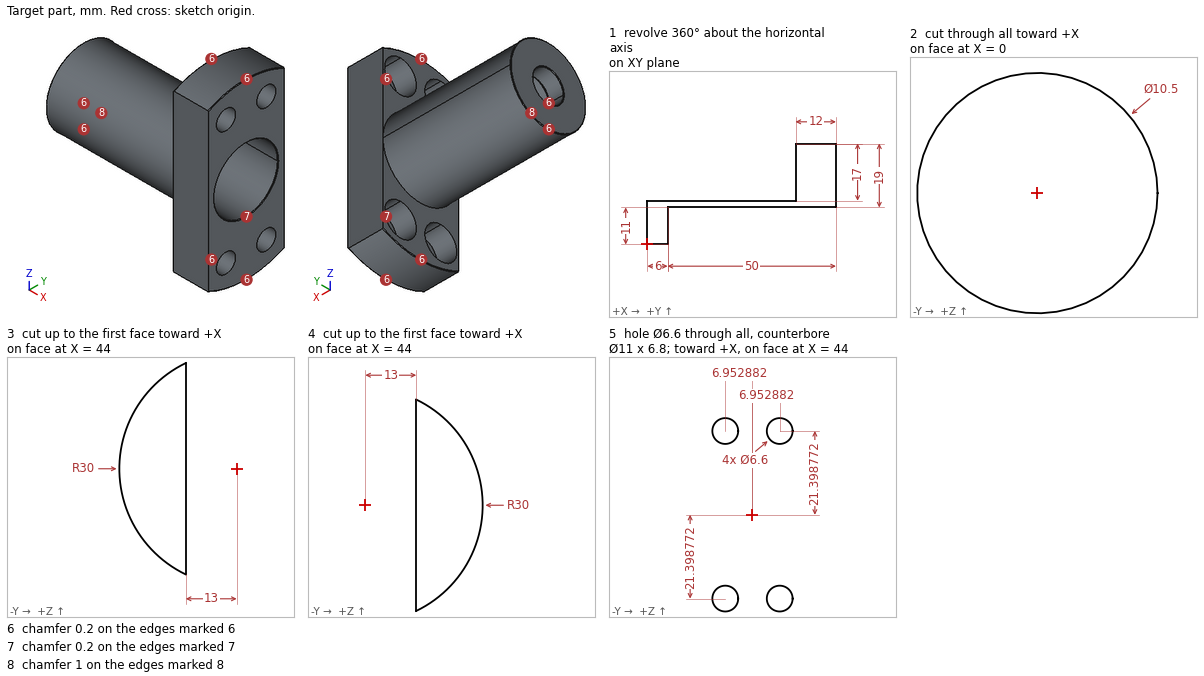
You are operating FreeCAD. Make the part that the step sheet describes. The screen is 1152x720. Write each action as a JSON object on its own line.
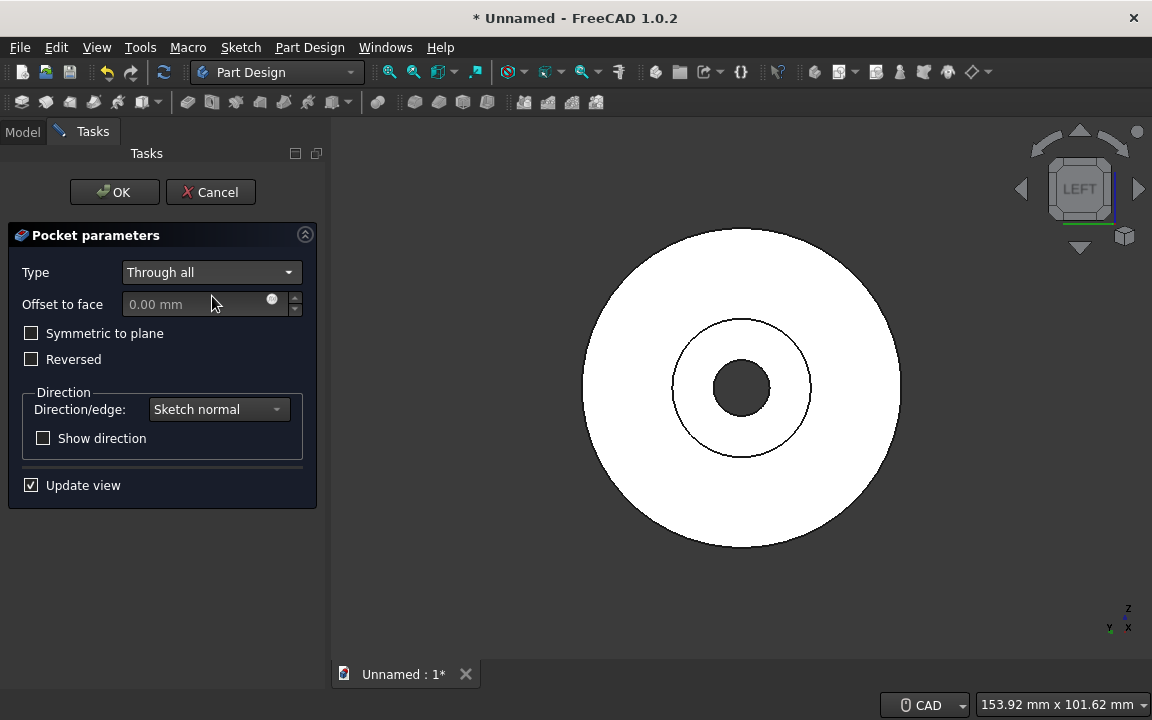
{"action": "left_click", "coordinate": [115, 192]}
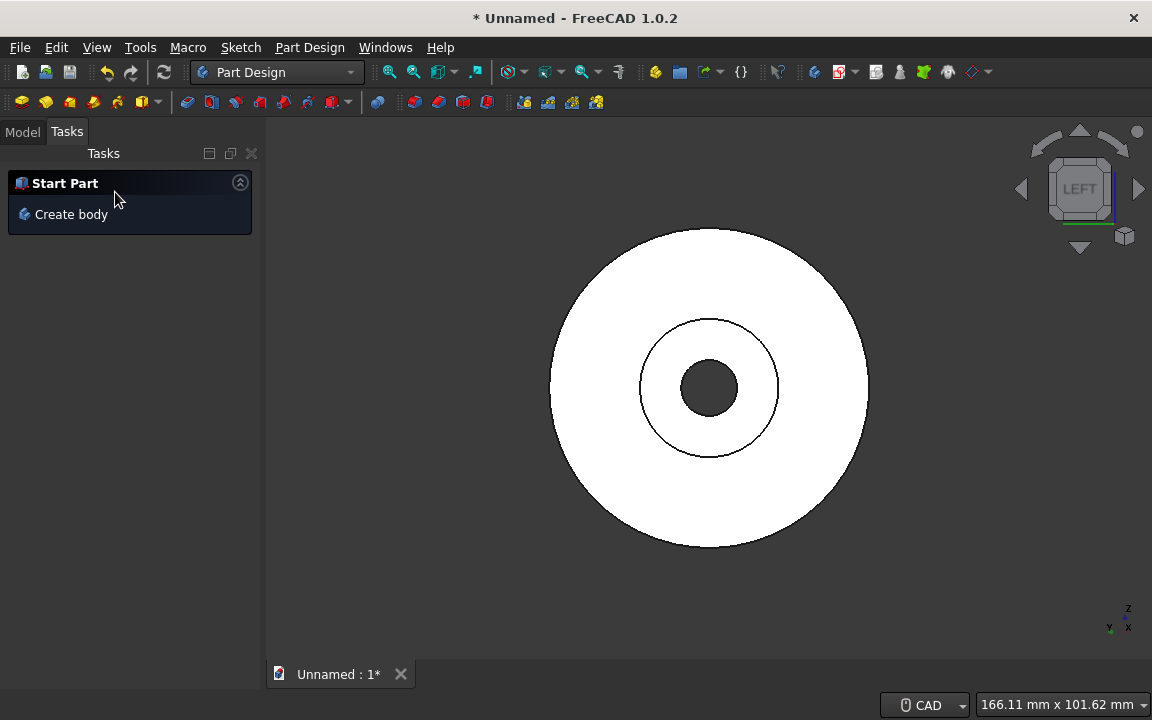
{"action": "left_click", "coordinate": [755, 296]}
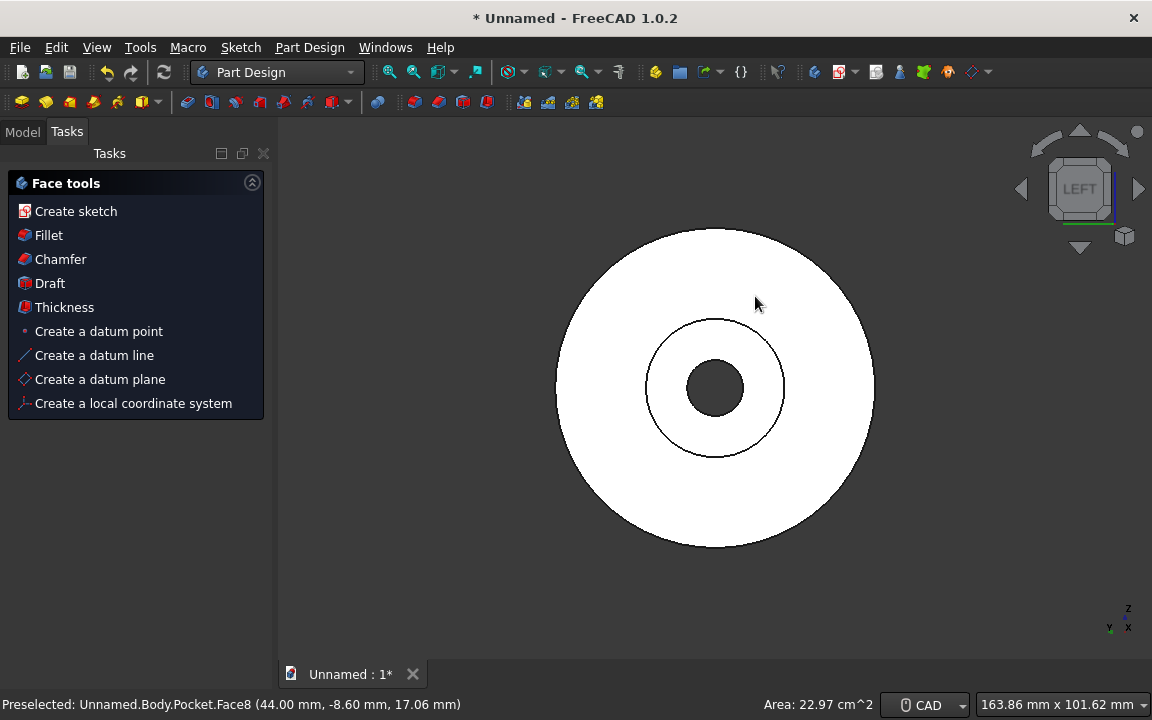
{"action": "left_click", "coordinate": [840, 72]}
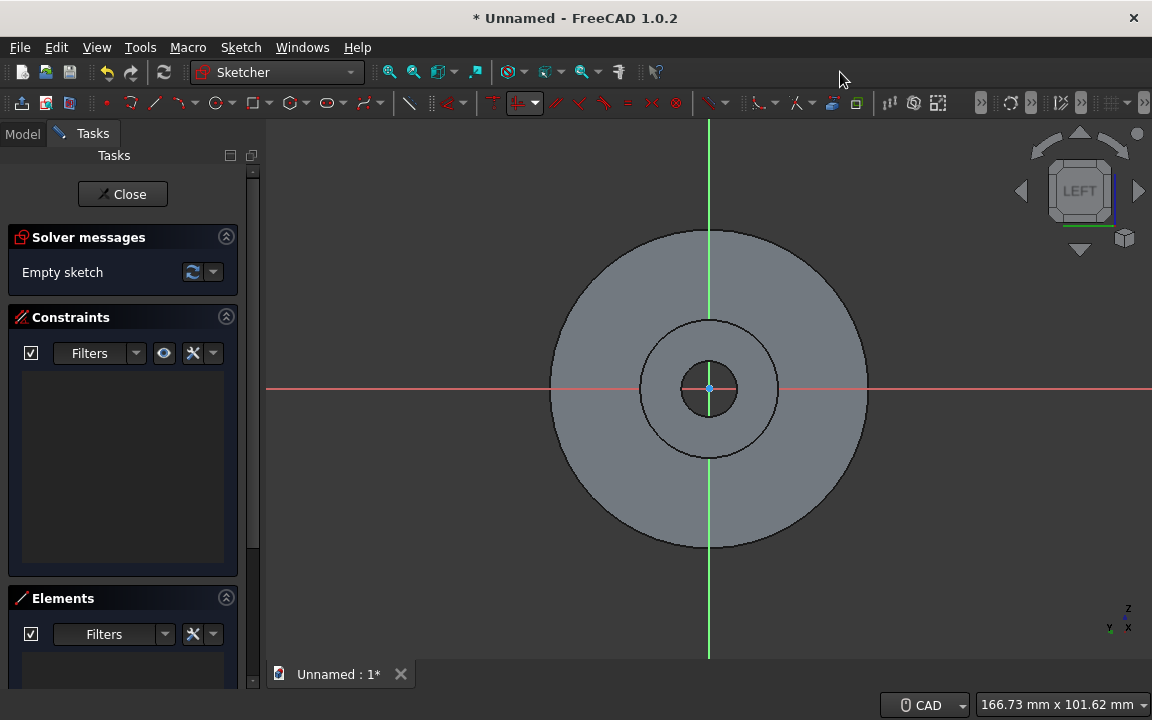
{"action": "left_click", "coordinate": [156, 104]}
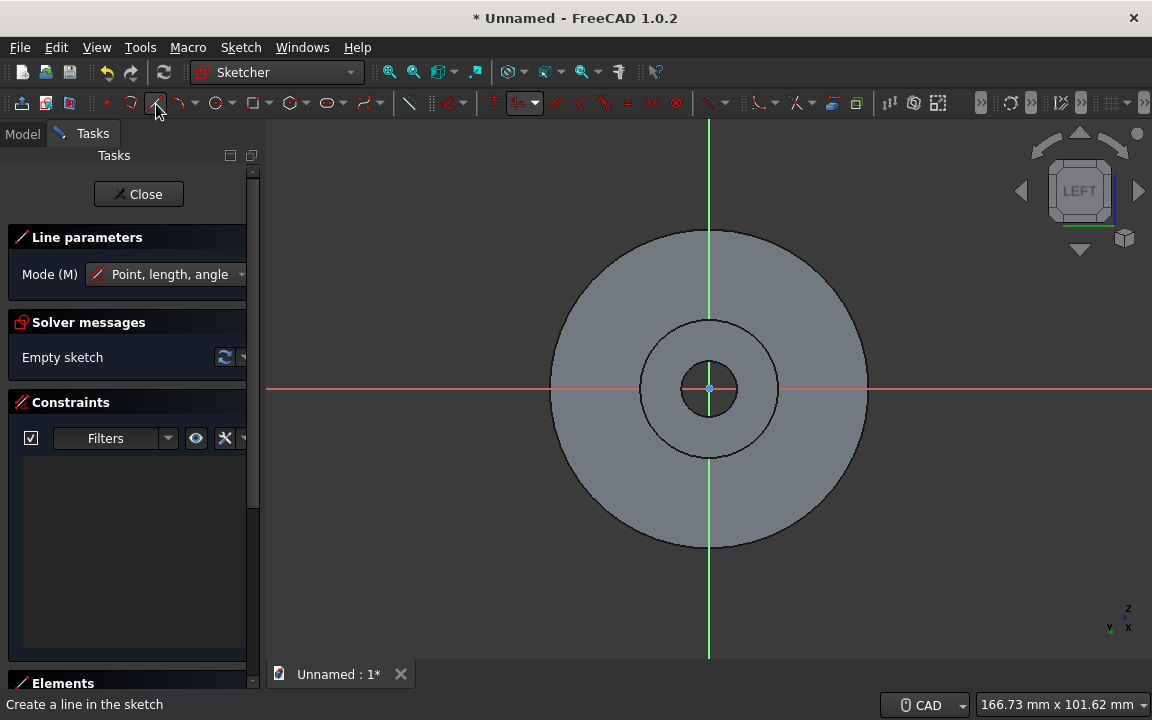
{"action": "left_click", "coordinate": [640, 533]}
{"action": "left_click", "coordinate": [640, 245]}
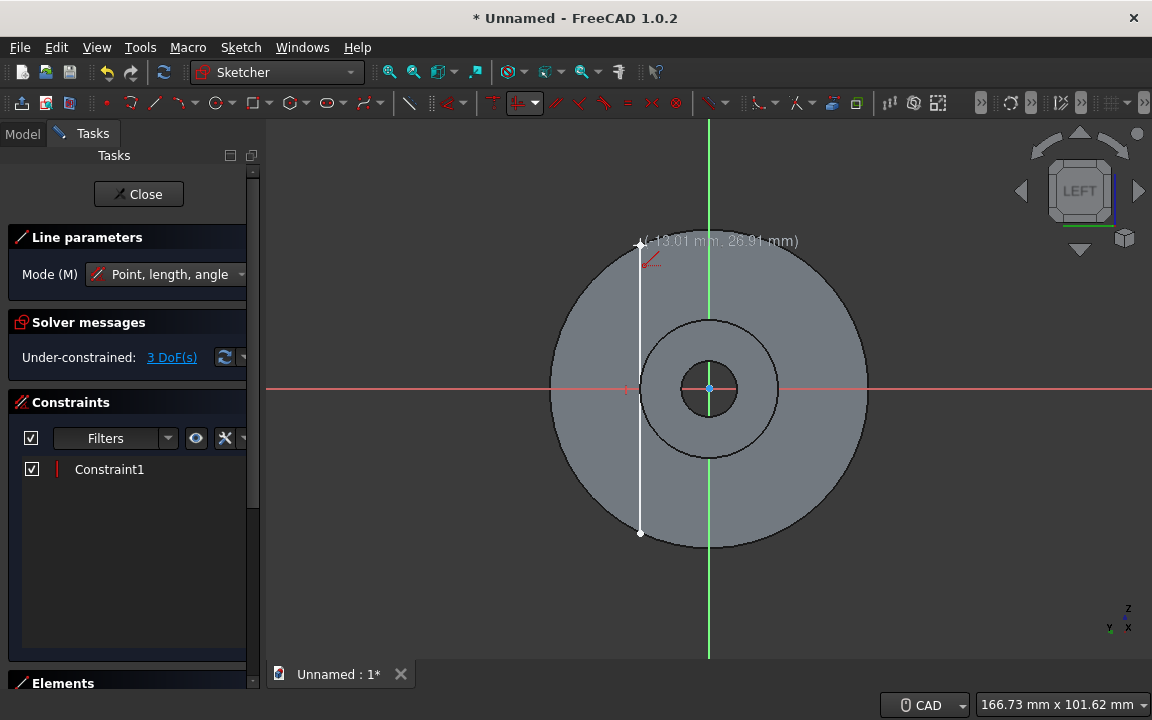
{"action": "left_click", "coordinate": [180, 104]}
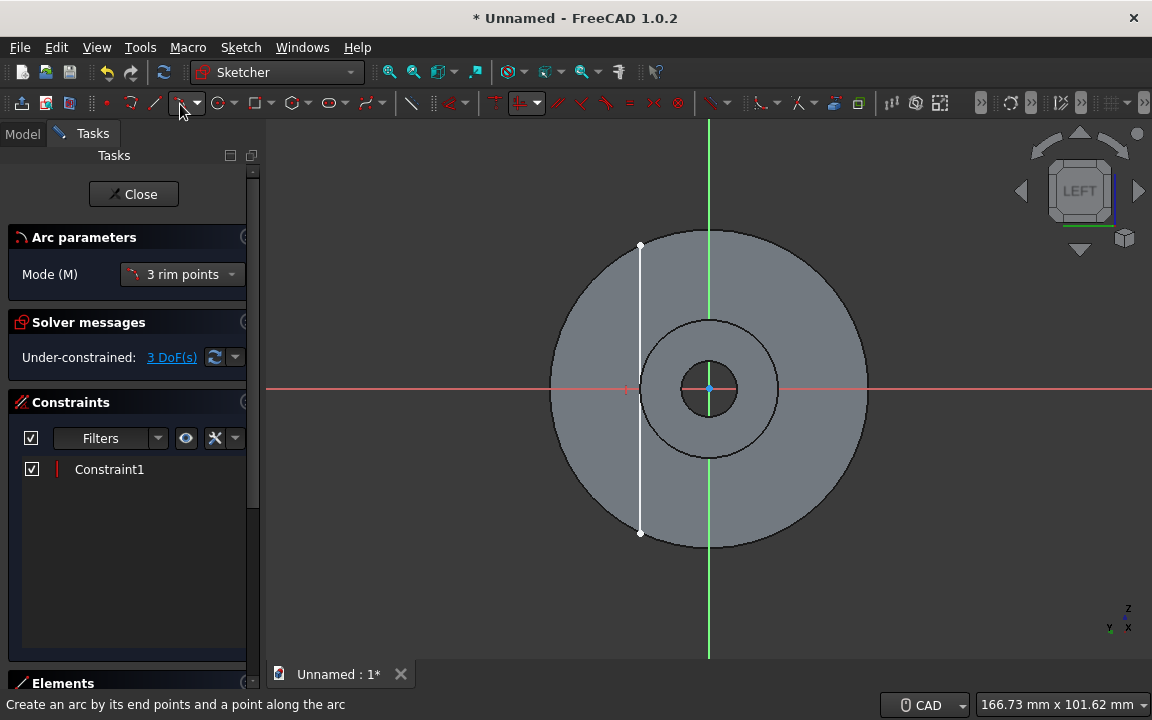
{"action": "left_click", "coordinate": [640, 246]}
{"action": "left_click", "coordinate": [640, 534]}
{"action": "left_click", "coordinate": [554, 354]}
{"action": "key", "text": "Escape"}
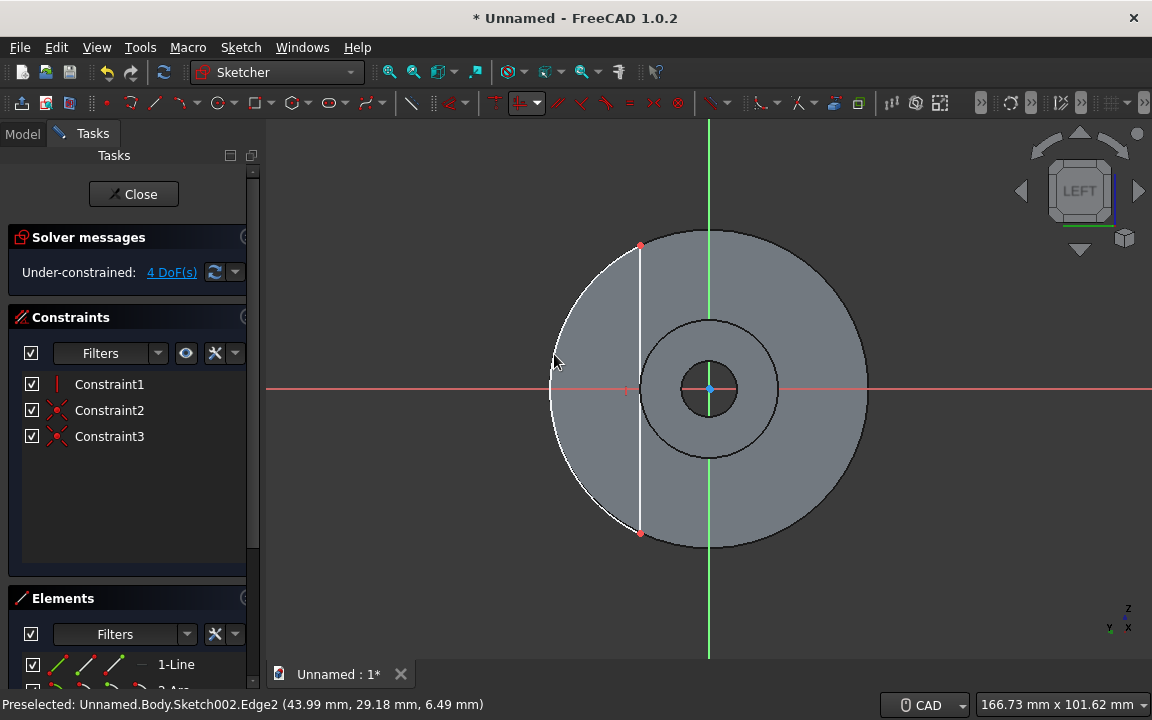
{"action": "left_click_drag", "start_coordinate": [699, 379], "coordinate": [720, 400]}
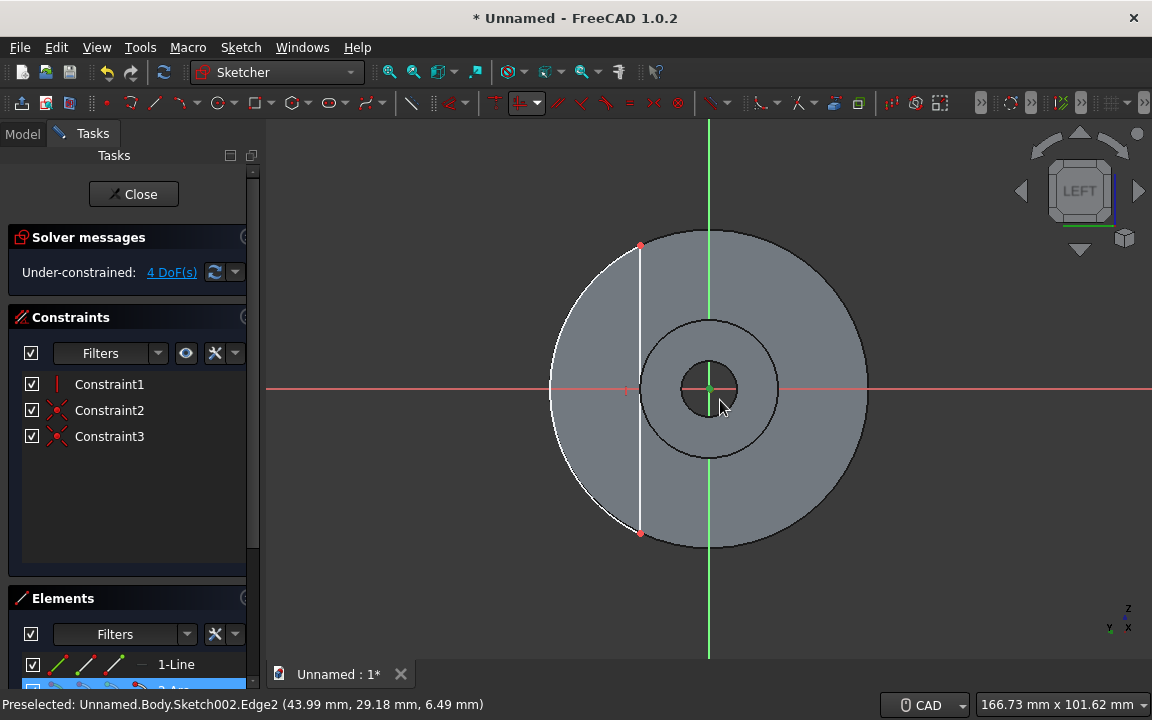
{"action": "left_click", "coordinate": [496, 104]}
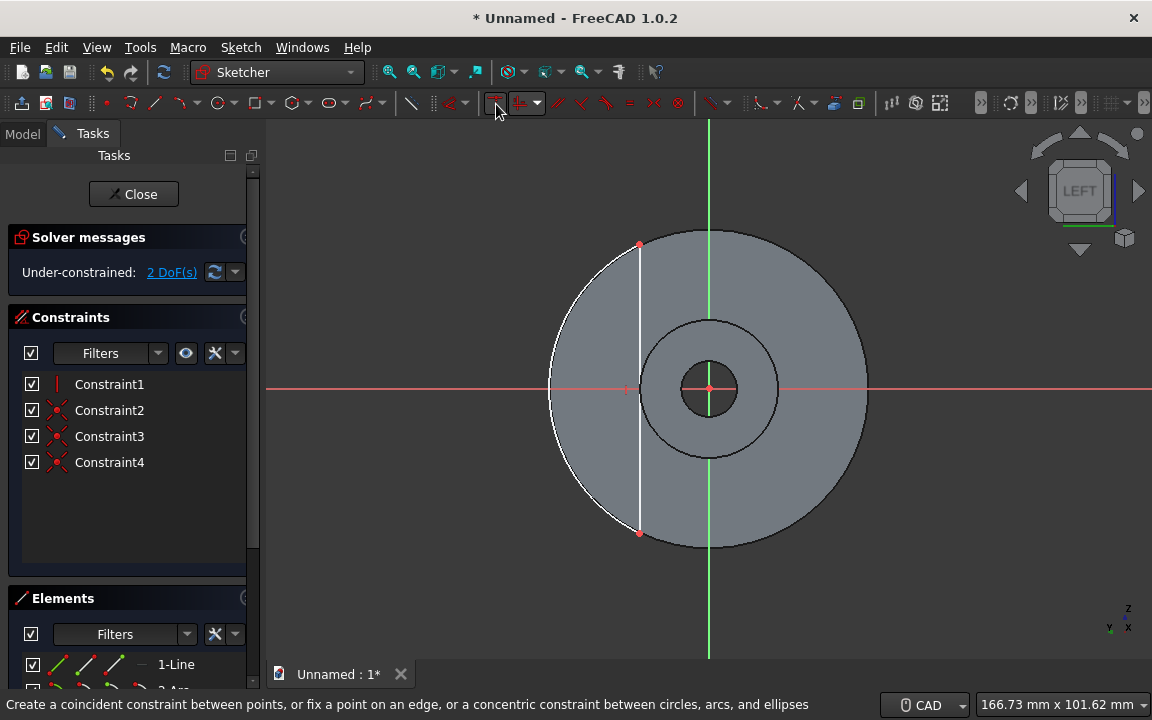
{"action": "left_click", "coordinate": [565, 319]}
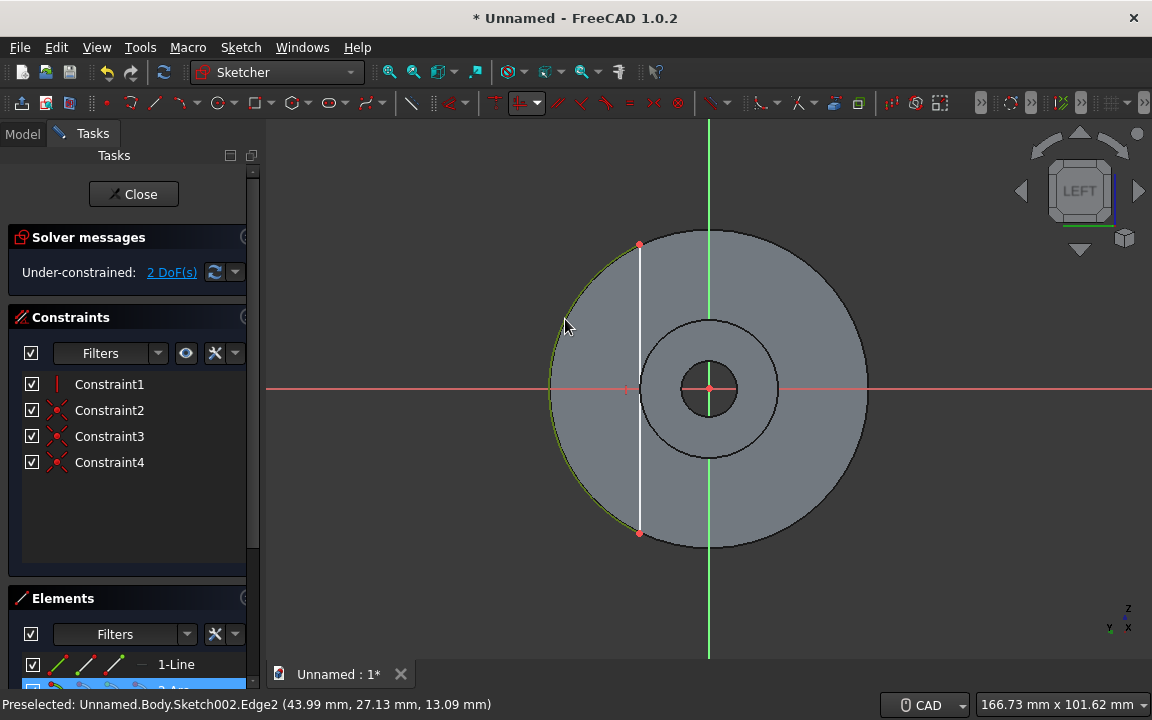
{"action": "key", "text": "k r"}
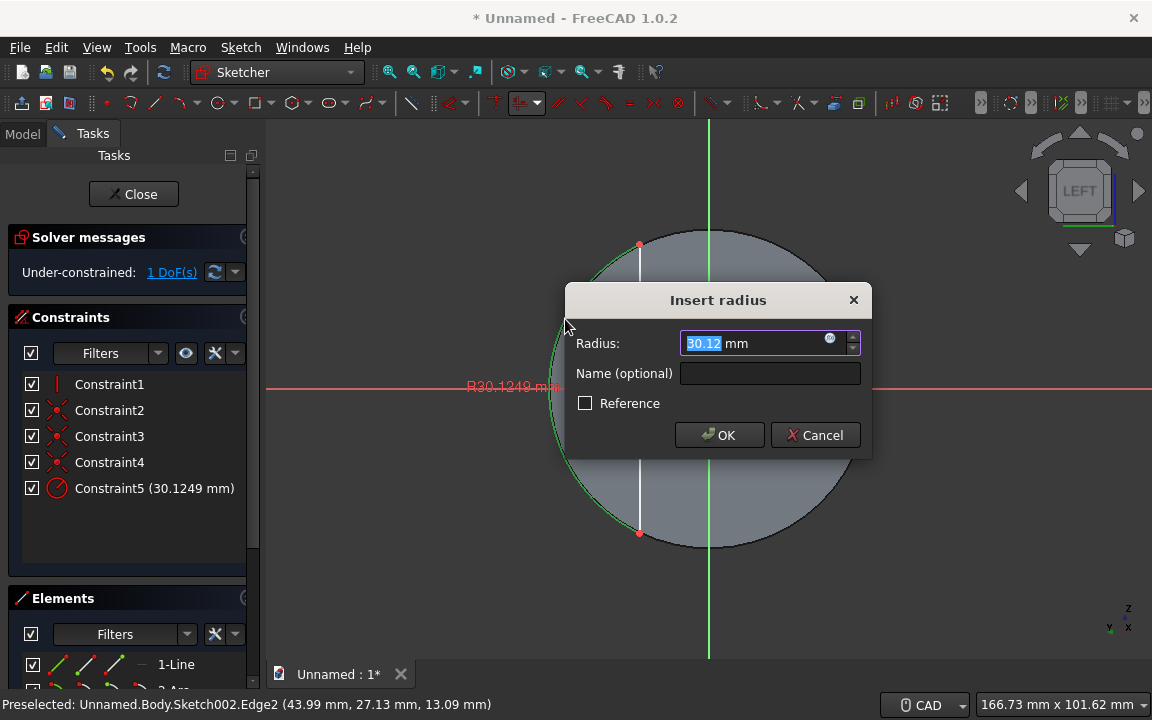
{"action": "type", "text": "30"}
{"action": "key", "text": "Return"}